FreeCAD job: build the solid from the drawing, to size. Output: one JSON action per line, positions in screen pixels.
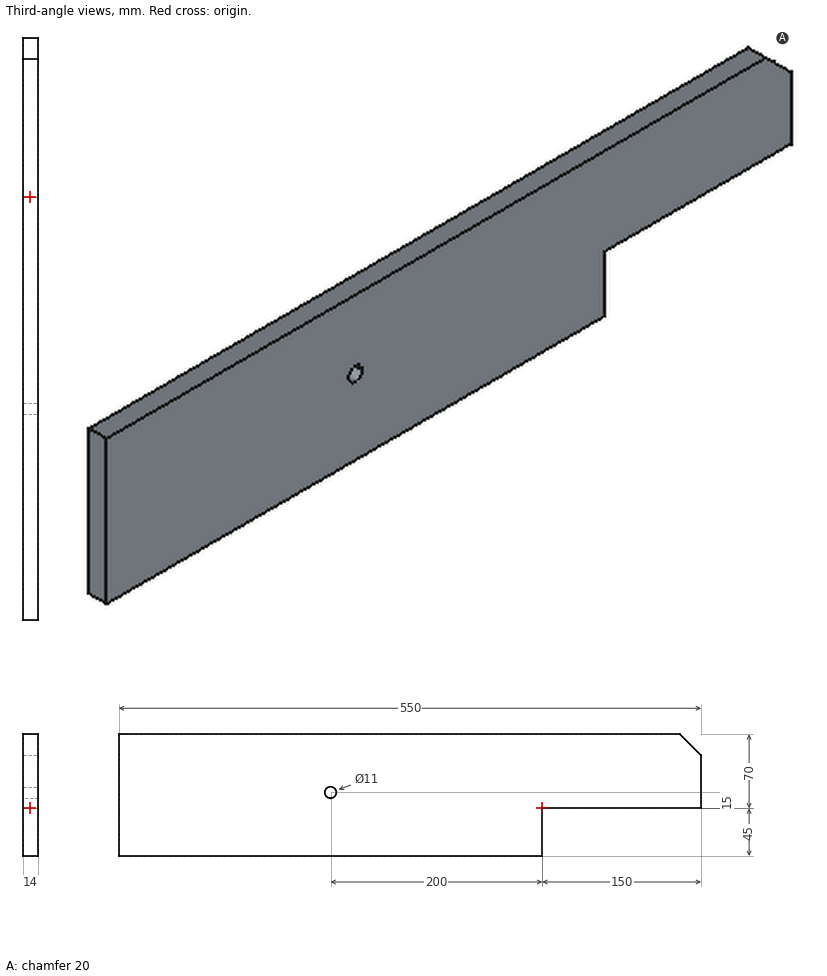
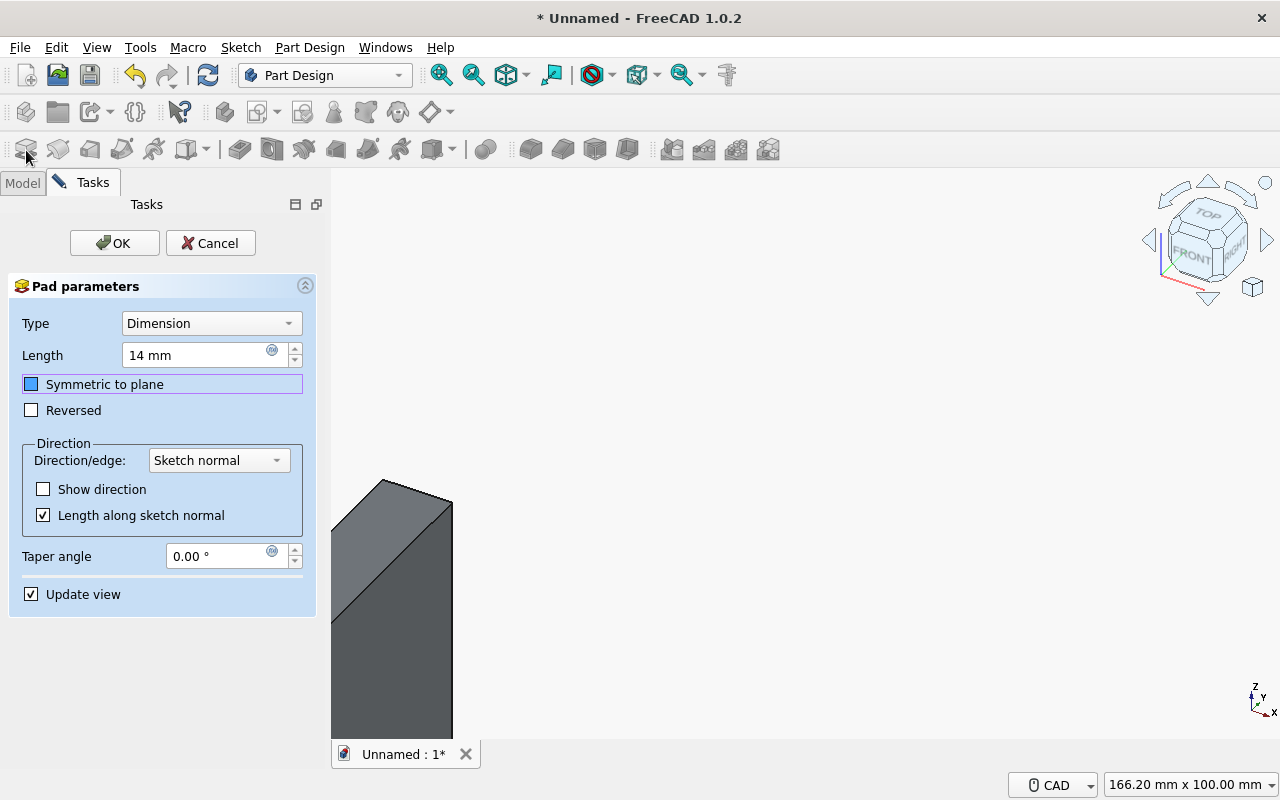
{"action": "left_click", "coordinate": [30, 384]}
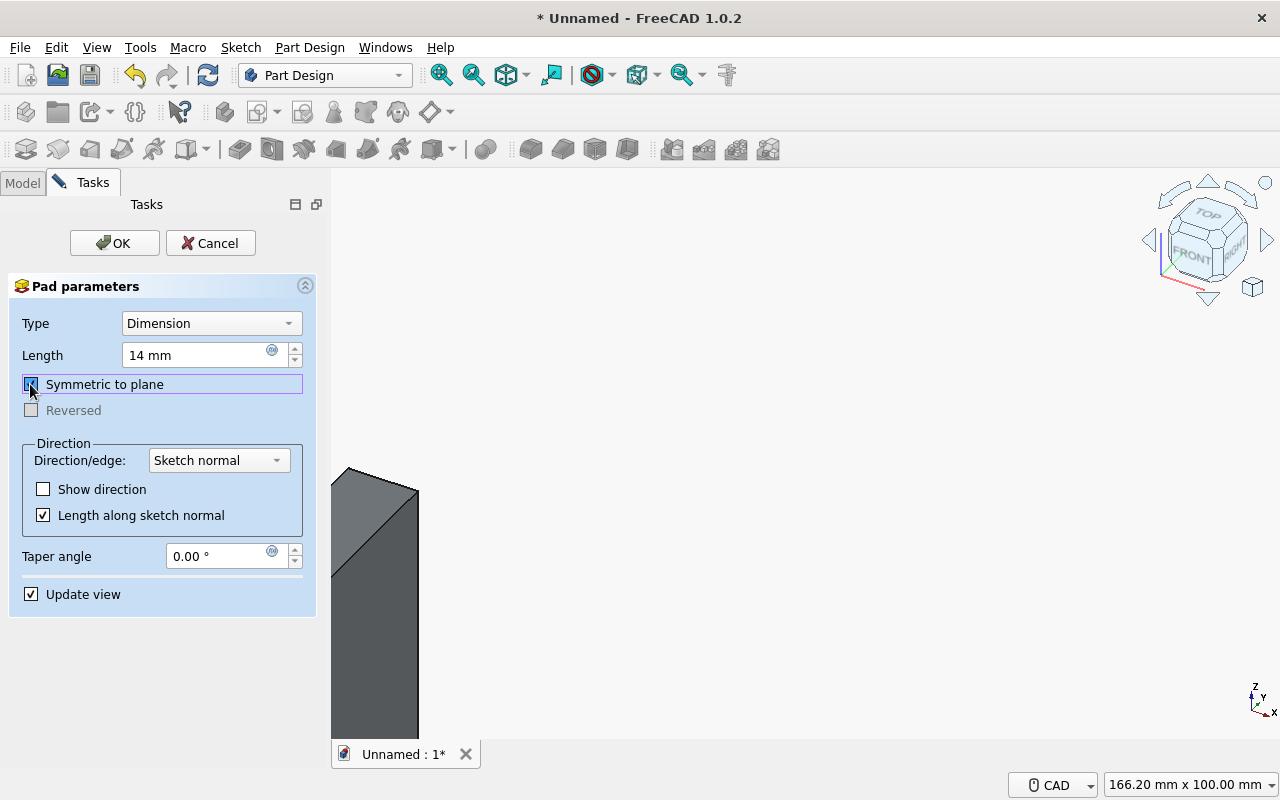
{"action": "left_click", "coordinate": [115, 243]}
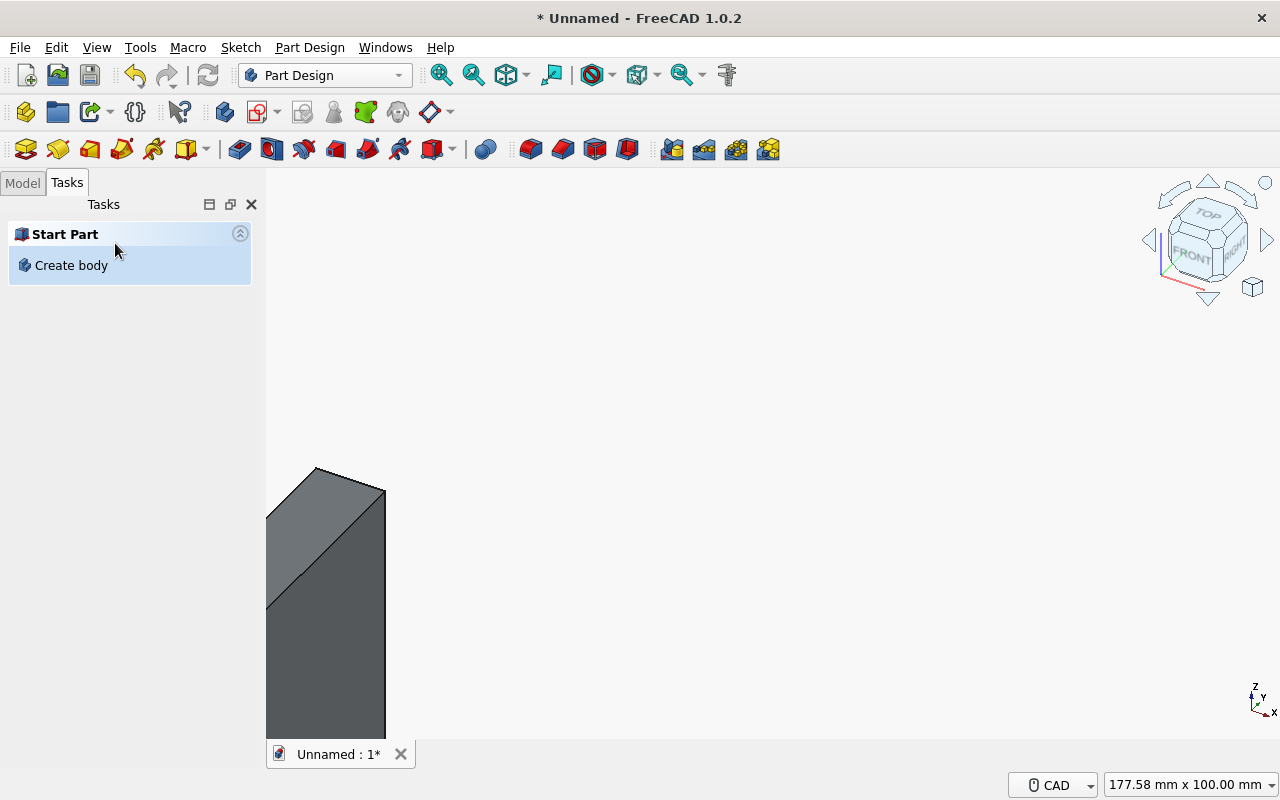
{"action": "left_click", "coordinate": [442, 76]}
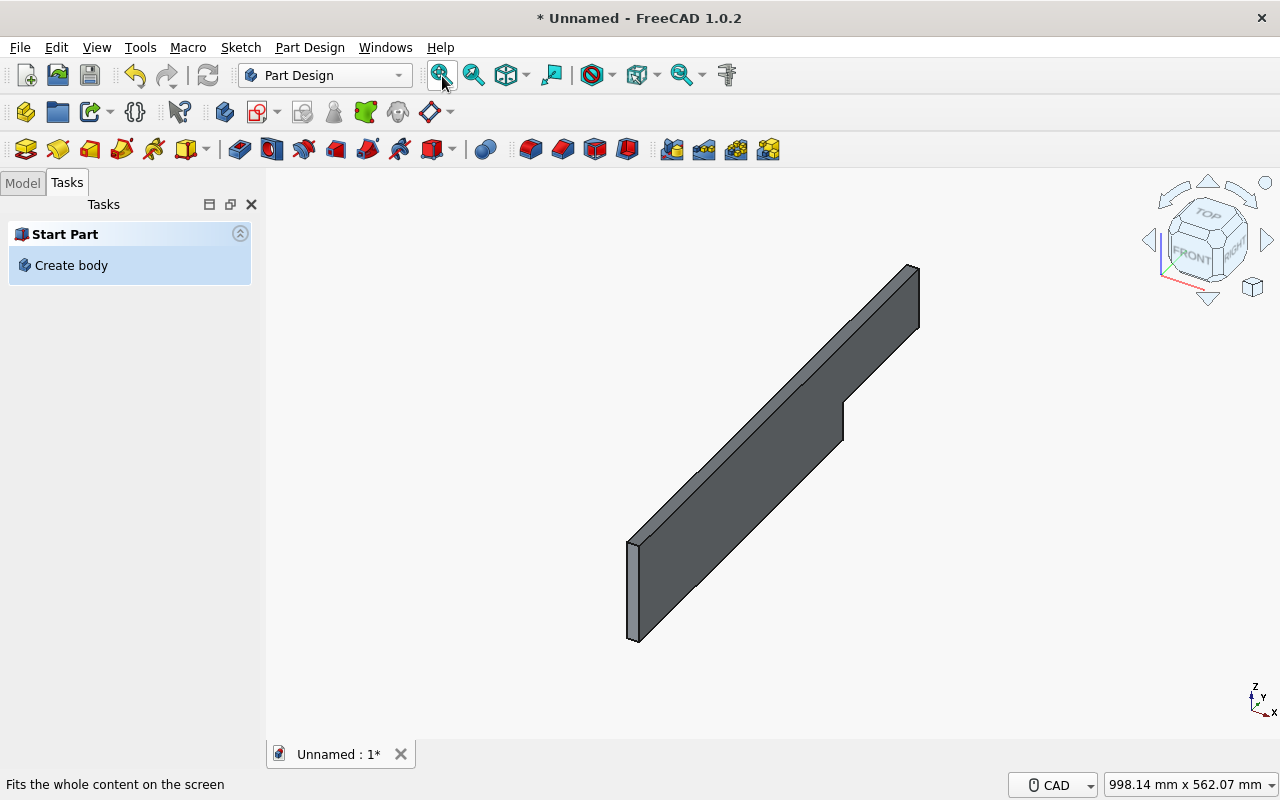
{"action": "left_click", "coordinate": [779, 455]}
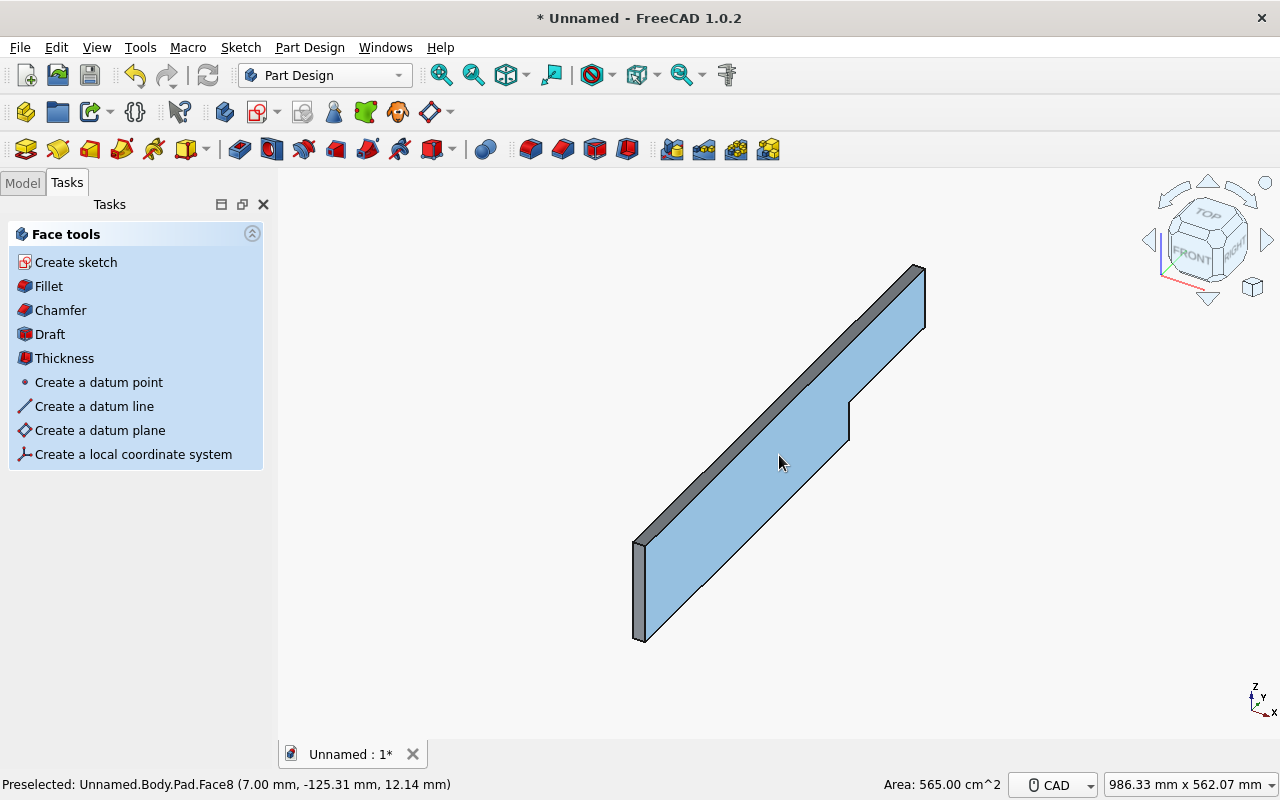
{"action": "left_click", "coordinate": [258, 112]}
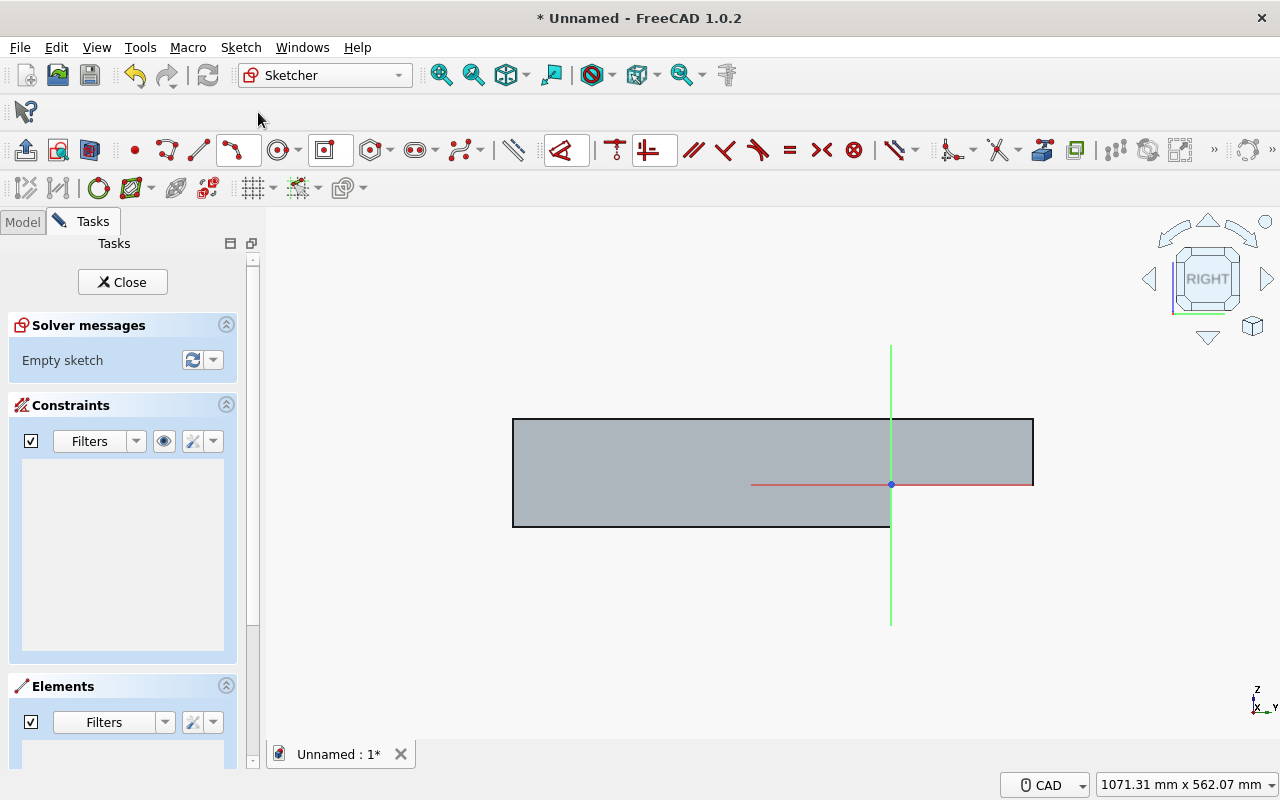
{"action": "scroll", "coordinate": [702, 471], "scroll_direction": "up", "scroll_amount": 15}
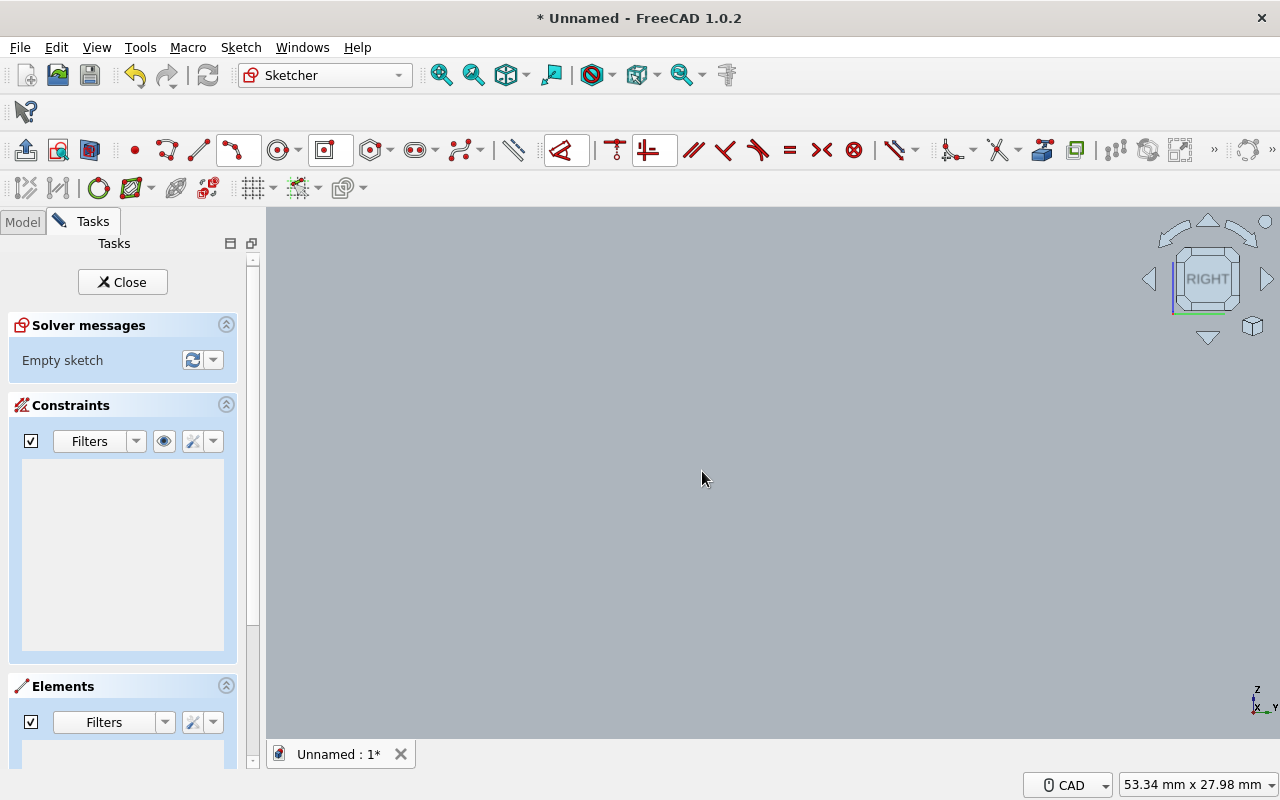
{"action": "scroll", "coordinate": [673, 416], "scroll_direction": "up", "scroll_amount": 2}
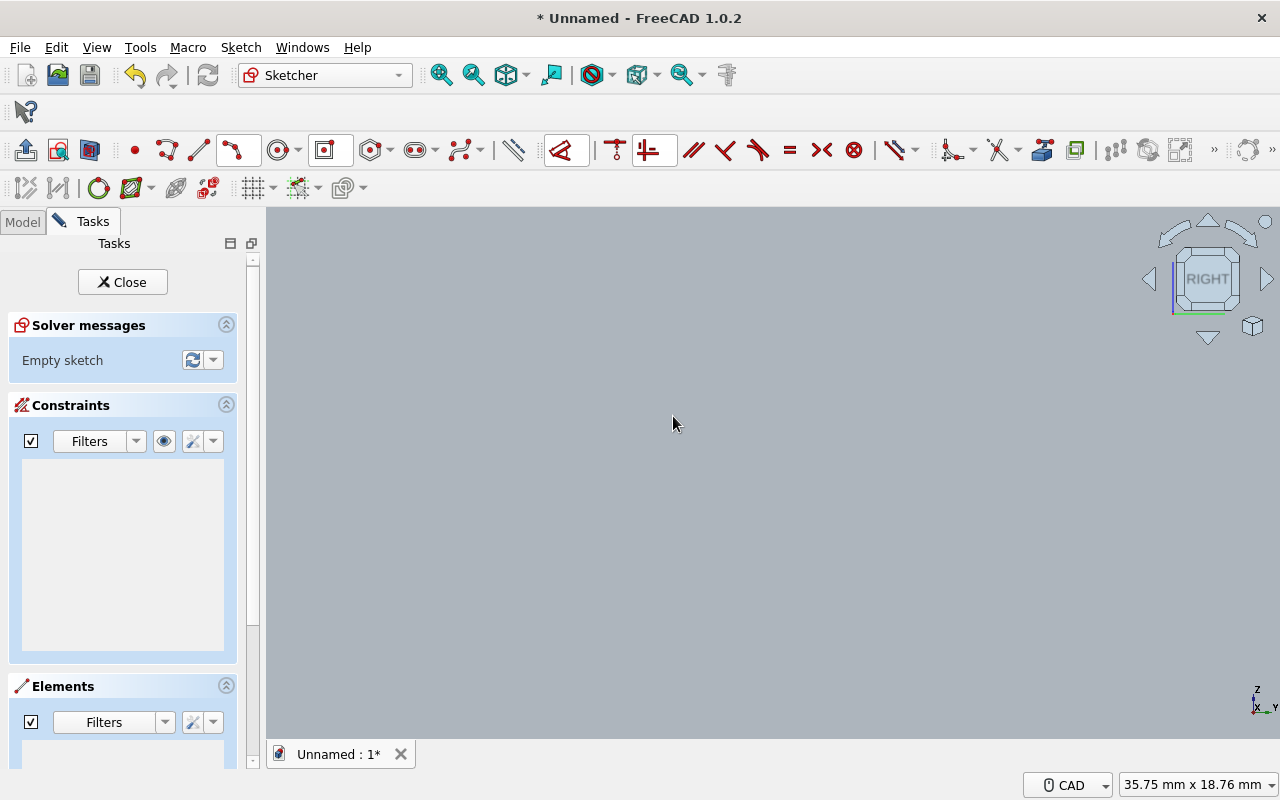
{"action": "left_click", "coordinate": [278, 150]}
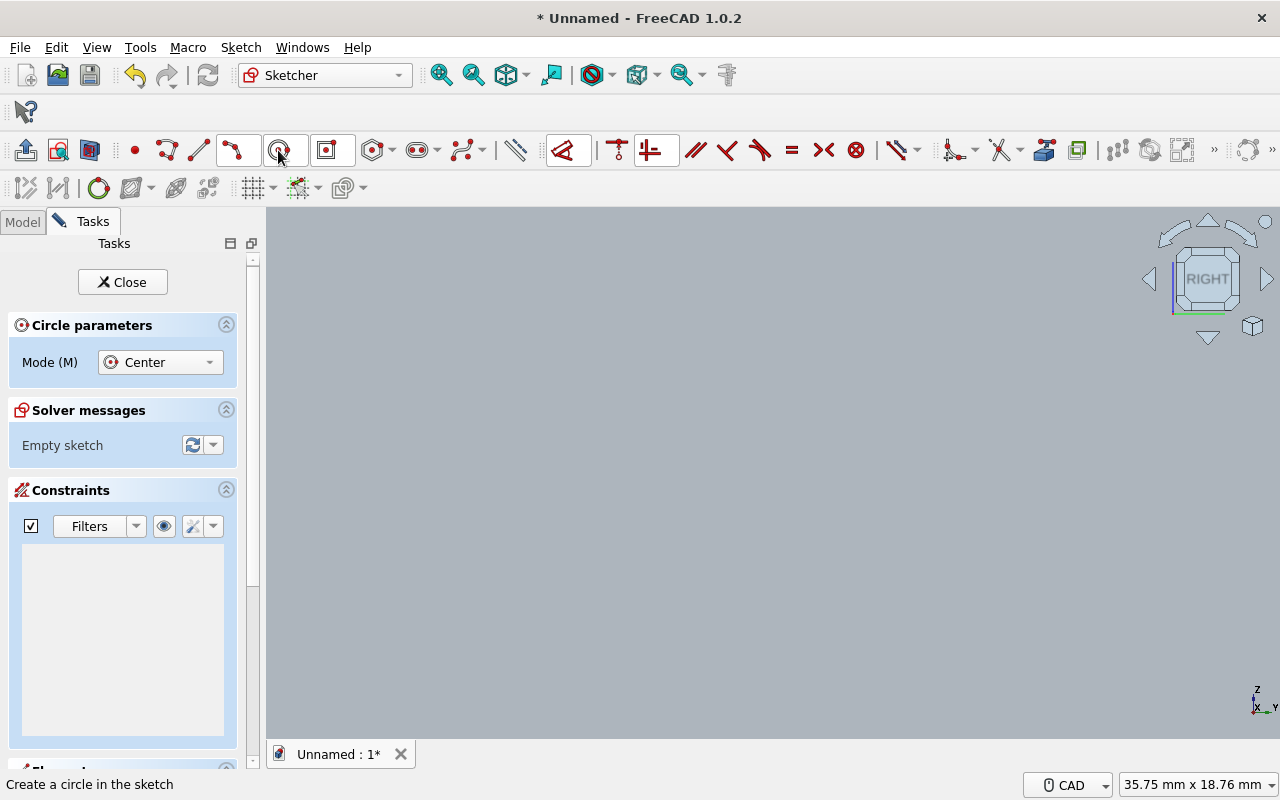
{"action": "left_click", "coordinate": [704, 473]}
{"action": "mouse_move", "coordinate": [814, 362]}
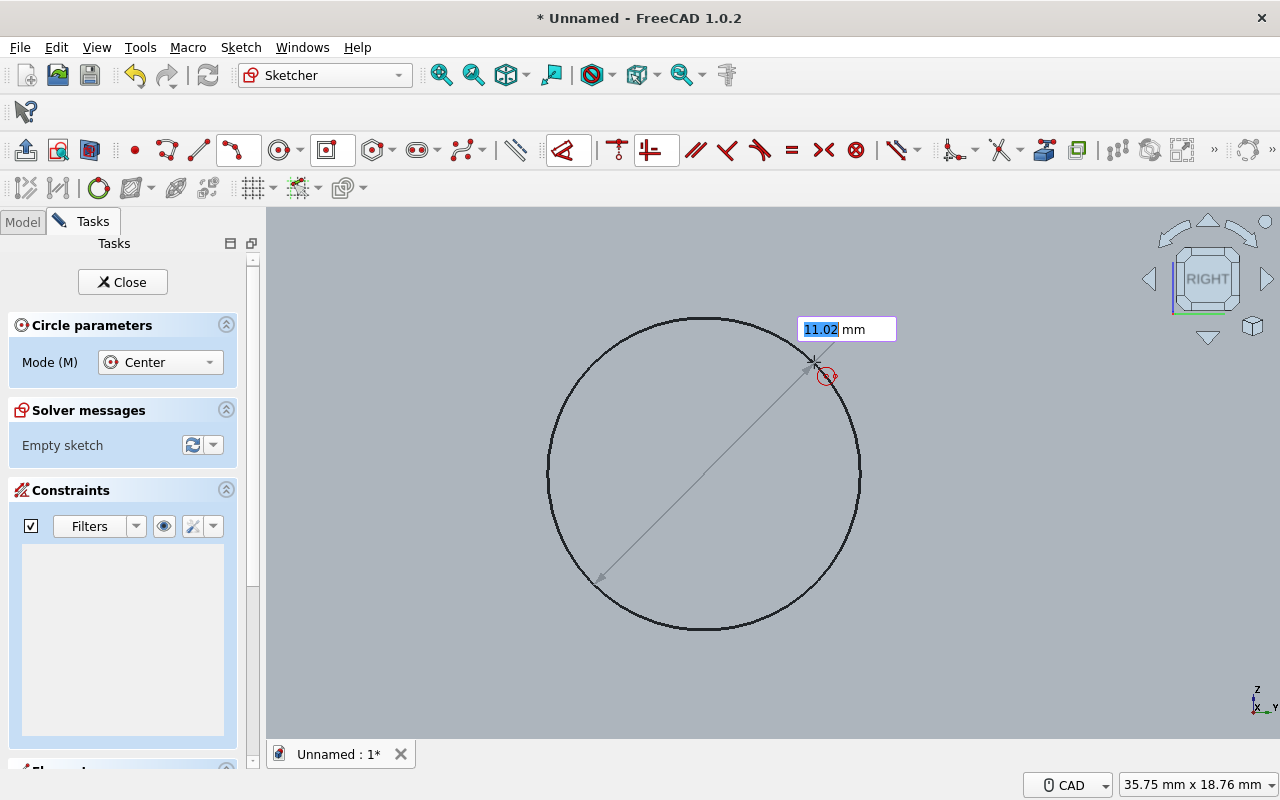
{"action": "type", "text": "11"}
{"action": "key", "text": "Return"}
{"action": "key", "text": "Escape"}